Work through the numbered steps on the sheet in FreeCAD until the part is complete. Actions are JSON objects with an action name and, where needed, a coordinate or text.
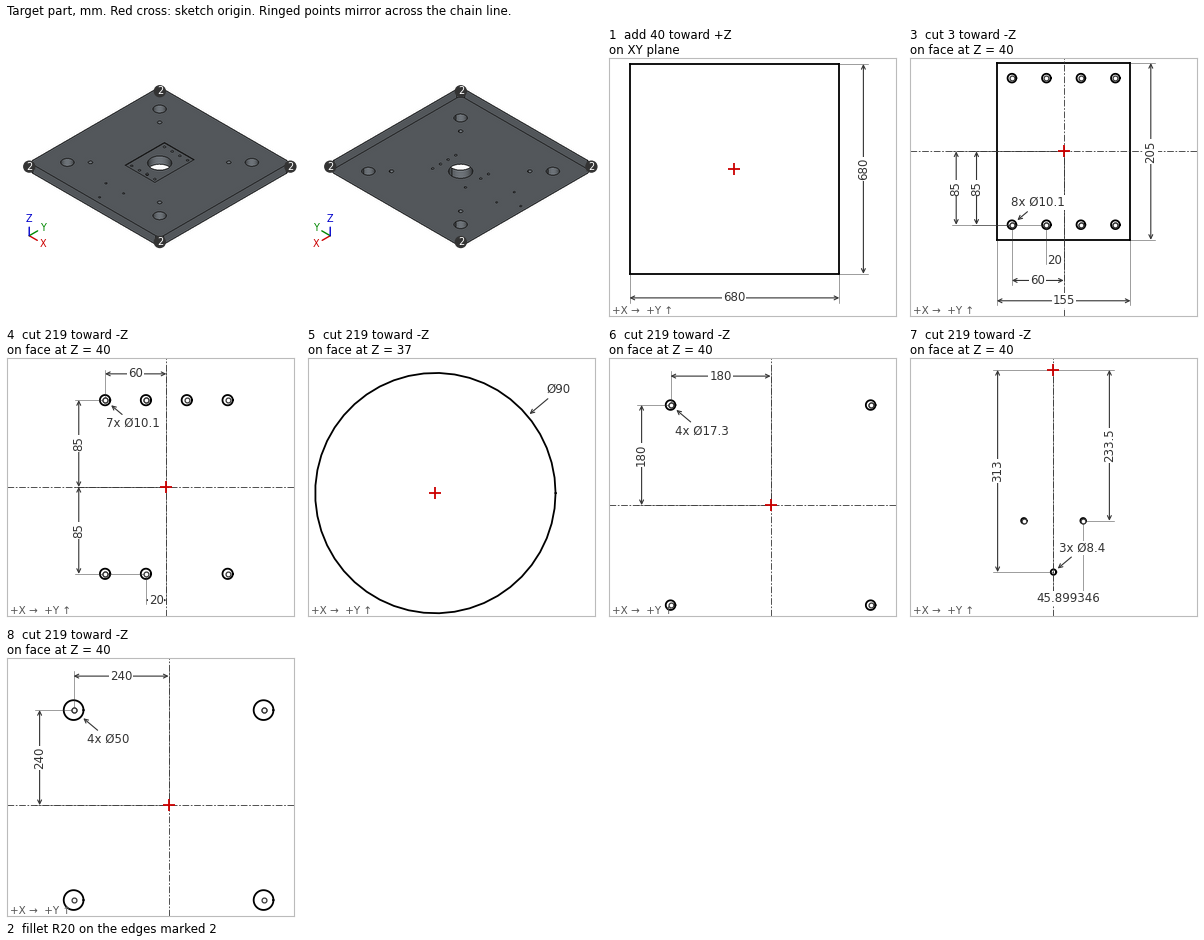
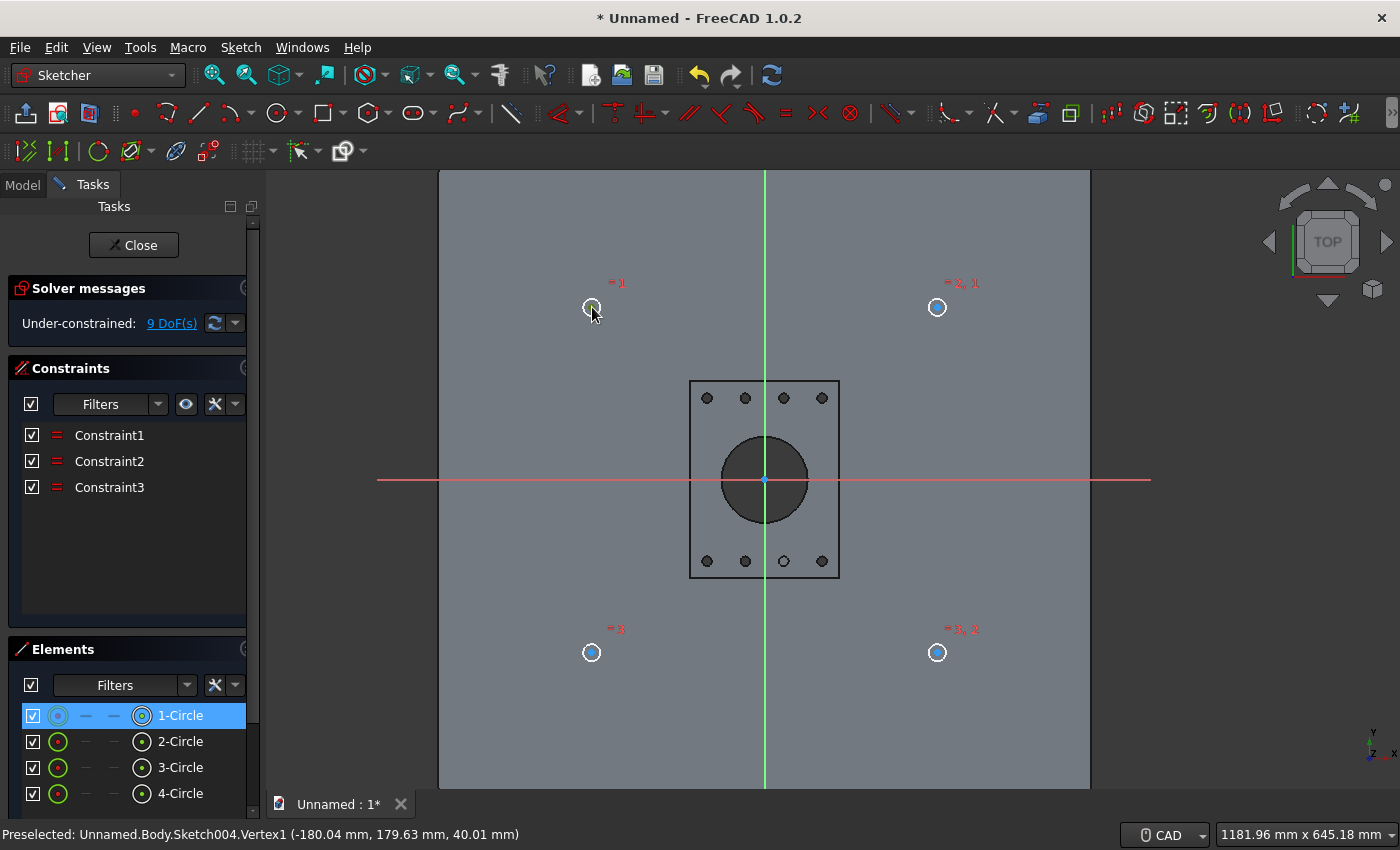
{"action": "left_click", "coordinate": [937, 307]}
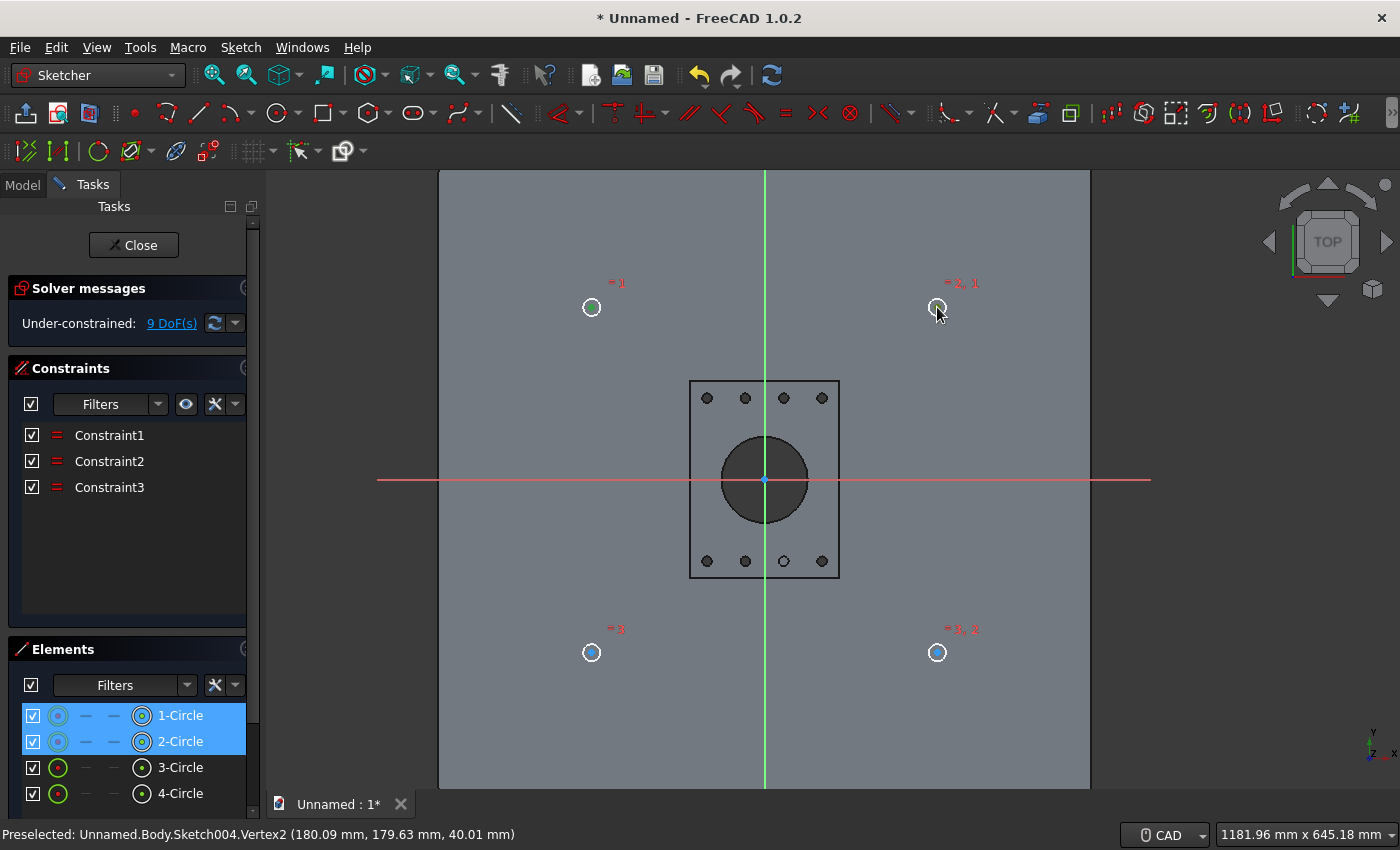
{"action": "left_click", "coordinate": [765, 721]}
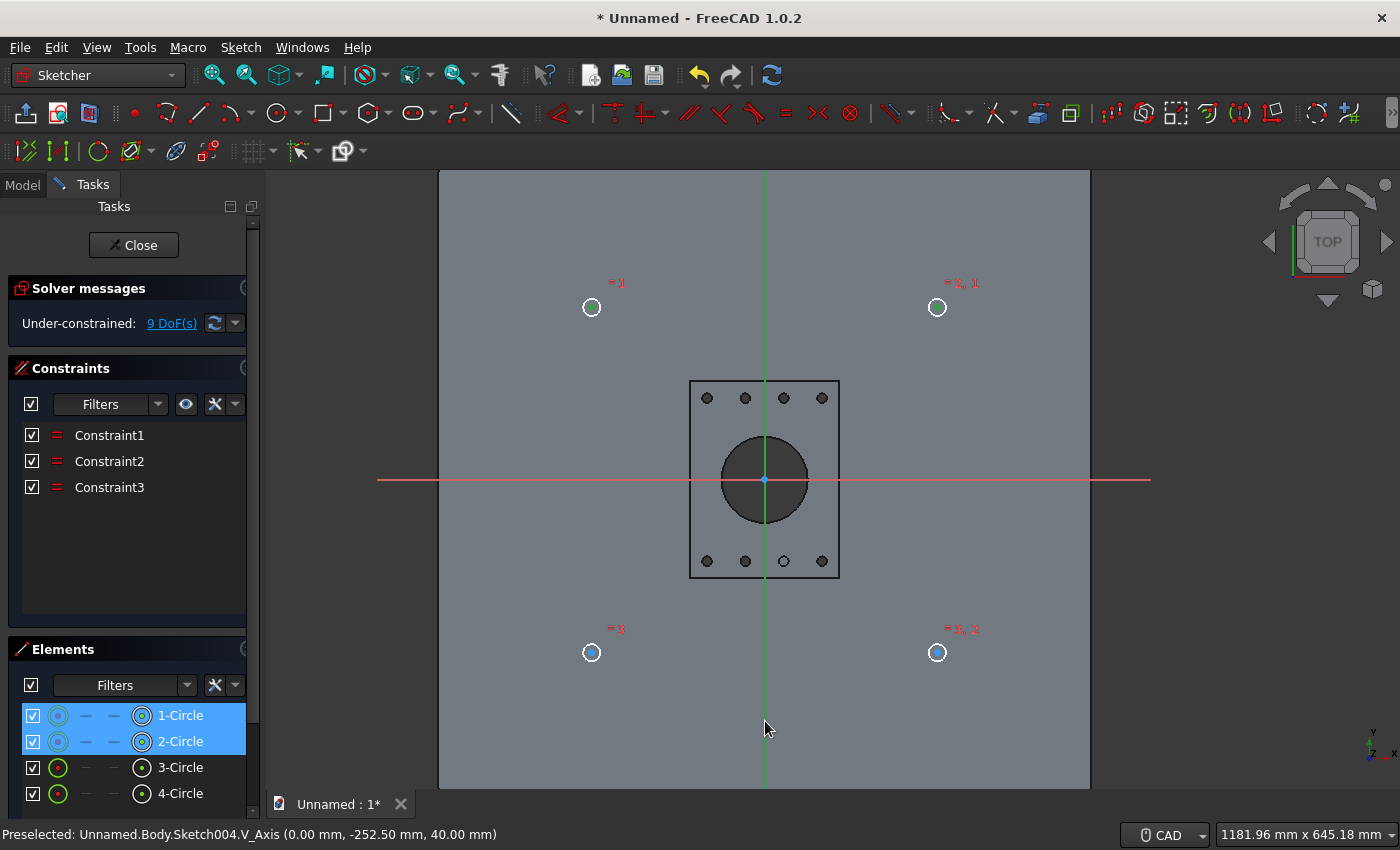
{"action": "left_click", "coordinate": [818, 114]}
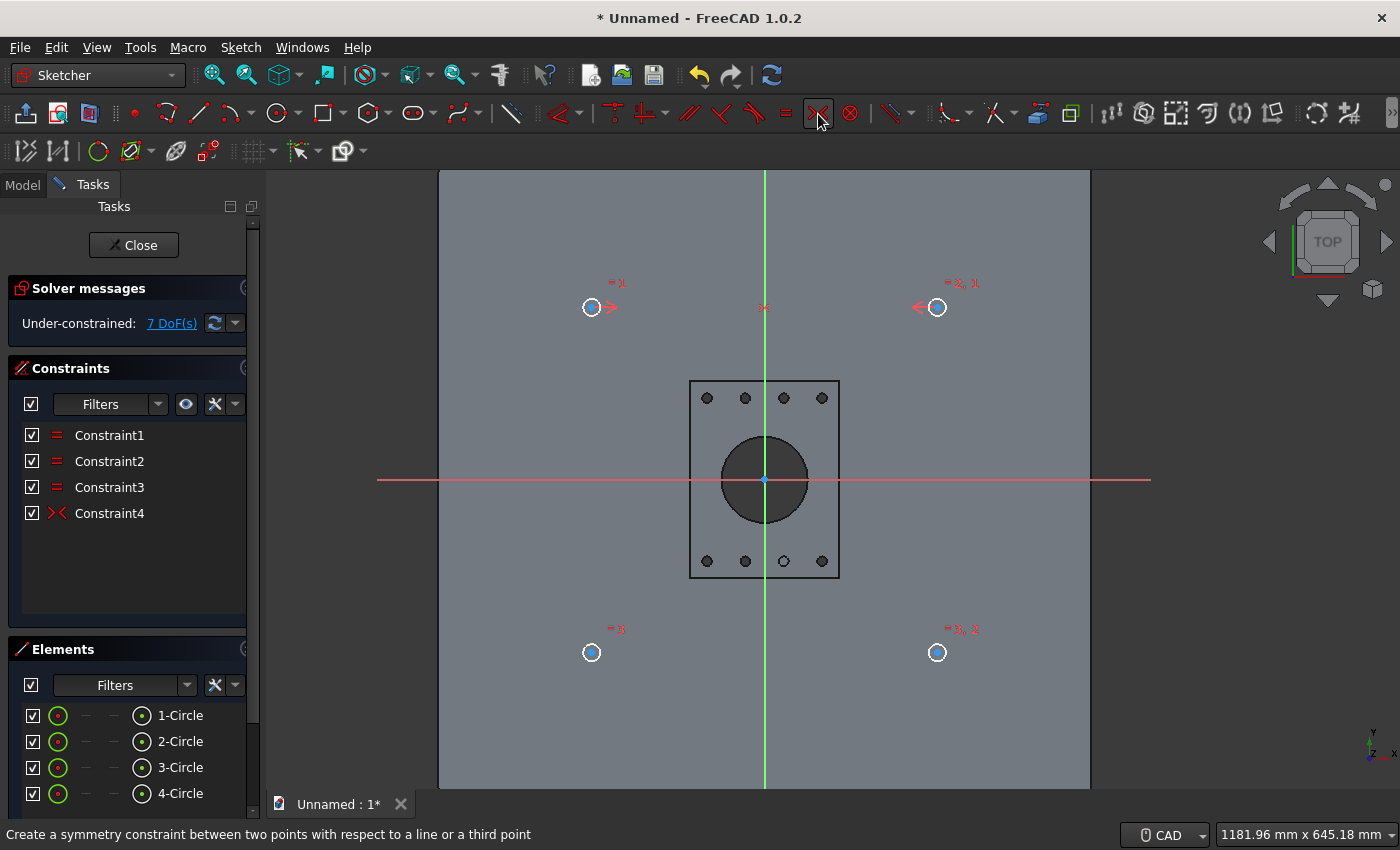
{"action": "left_click", "coordinate": [937, 307]}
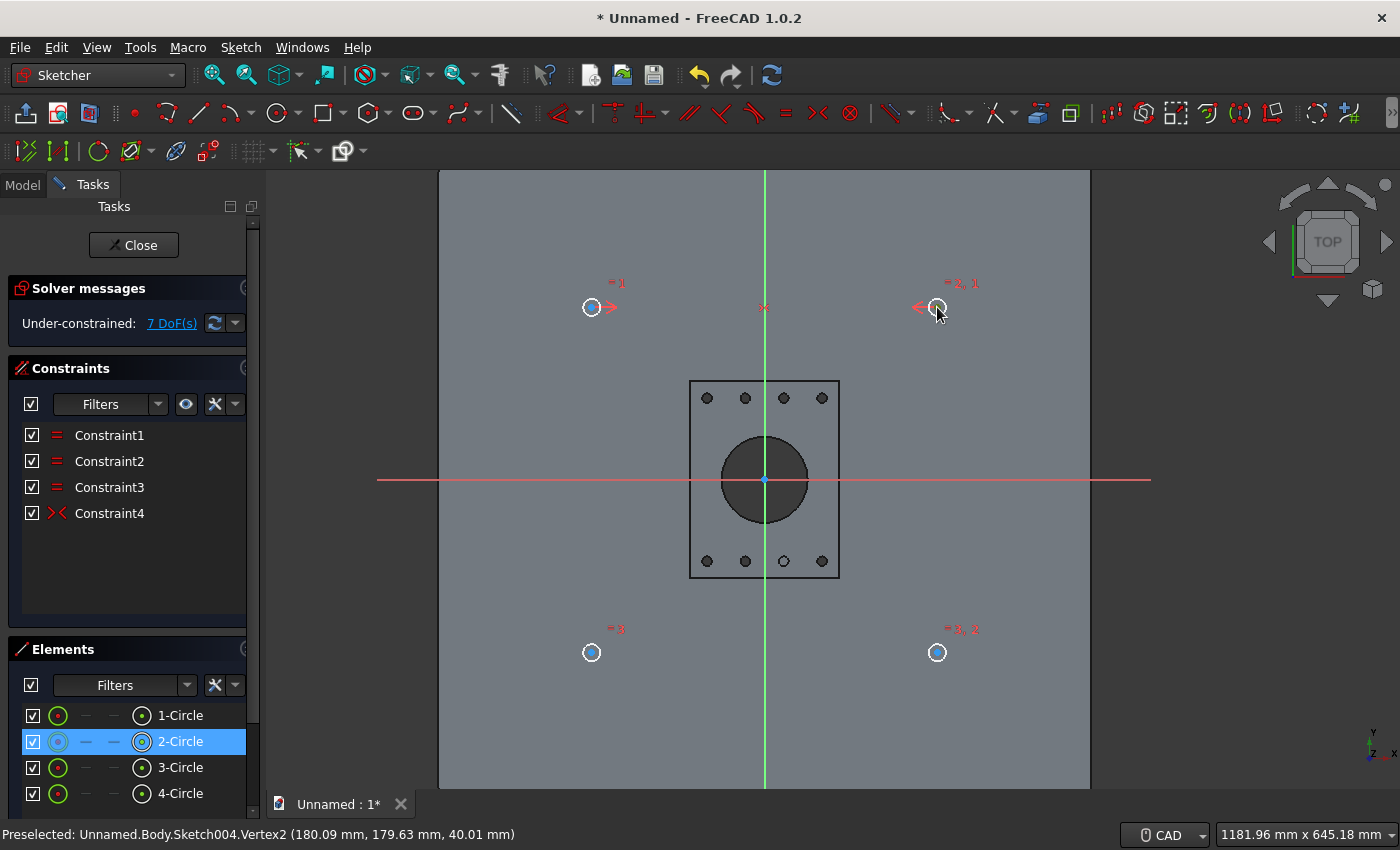
{"action": "left_click", "coordinate": [937, 653]}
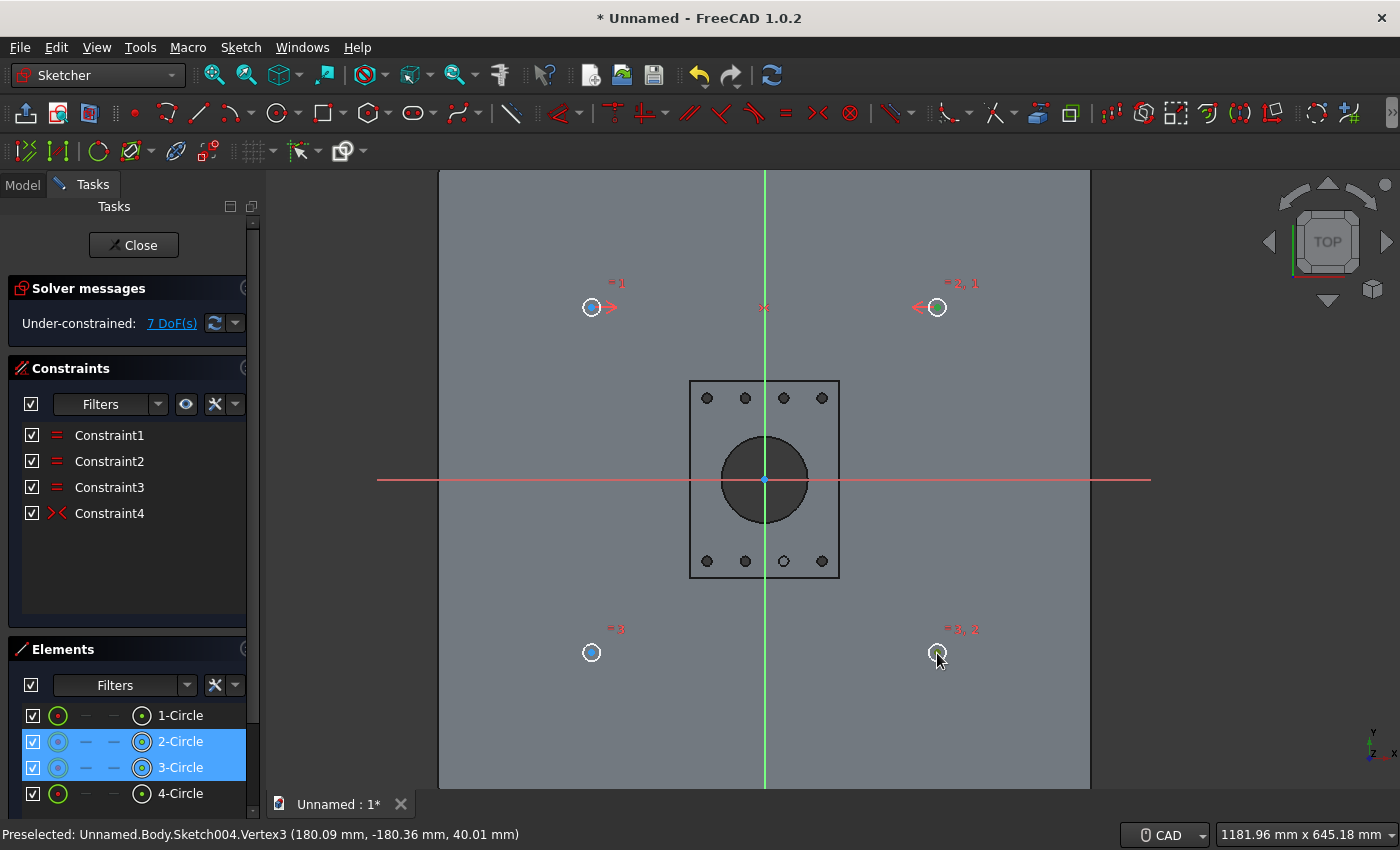
{"action": "left_click", "coordinate": [428, 480]}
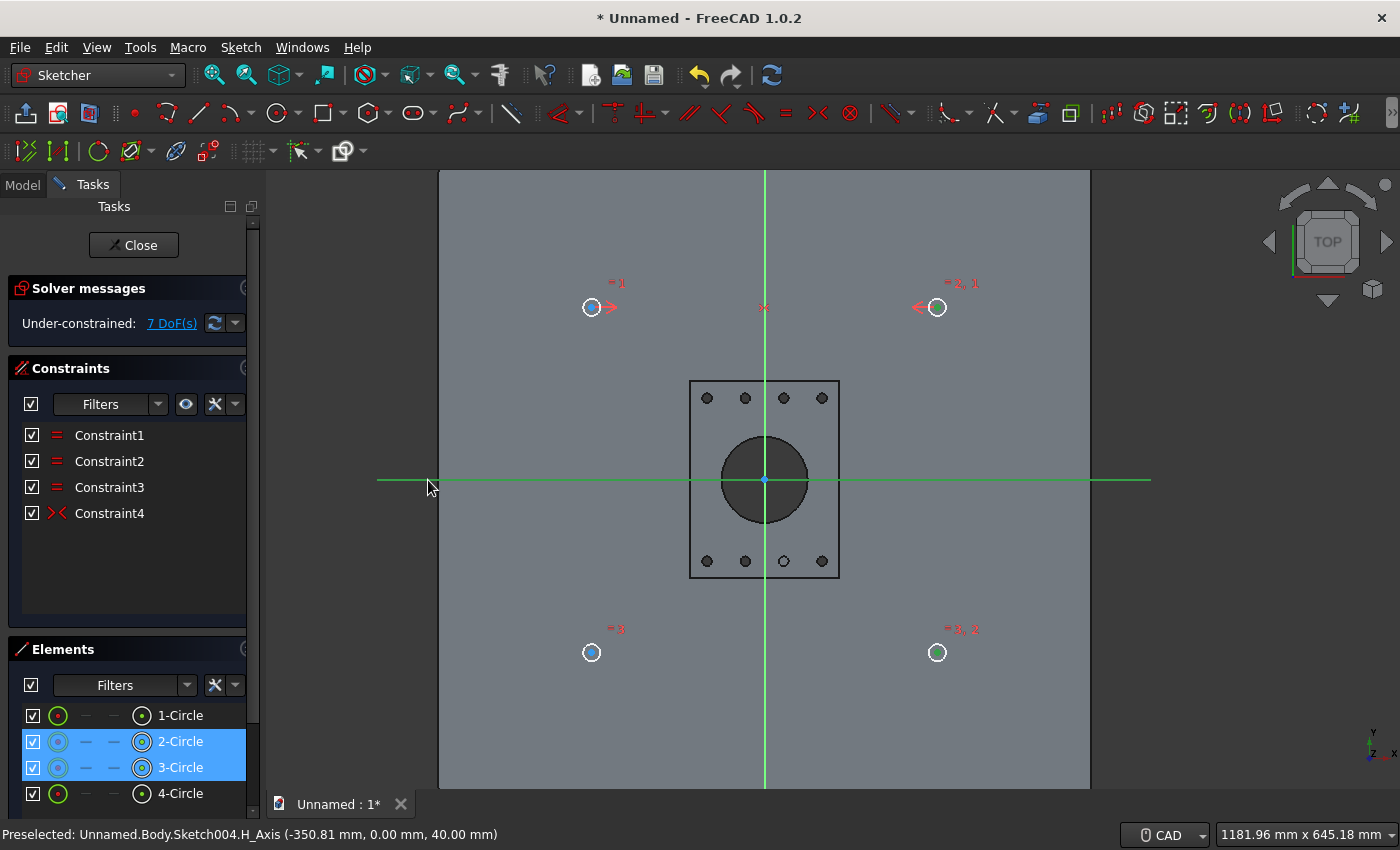
{"action": "left_click", "coordinate": [818, 114]}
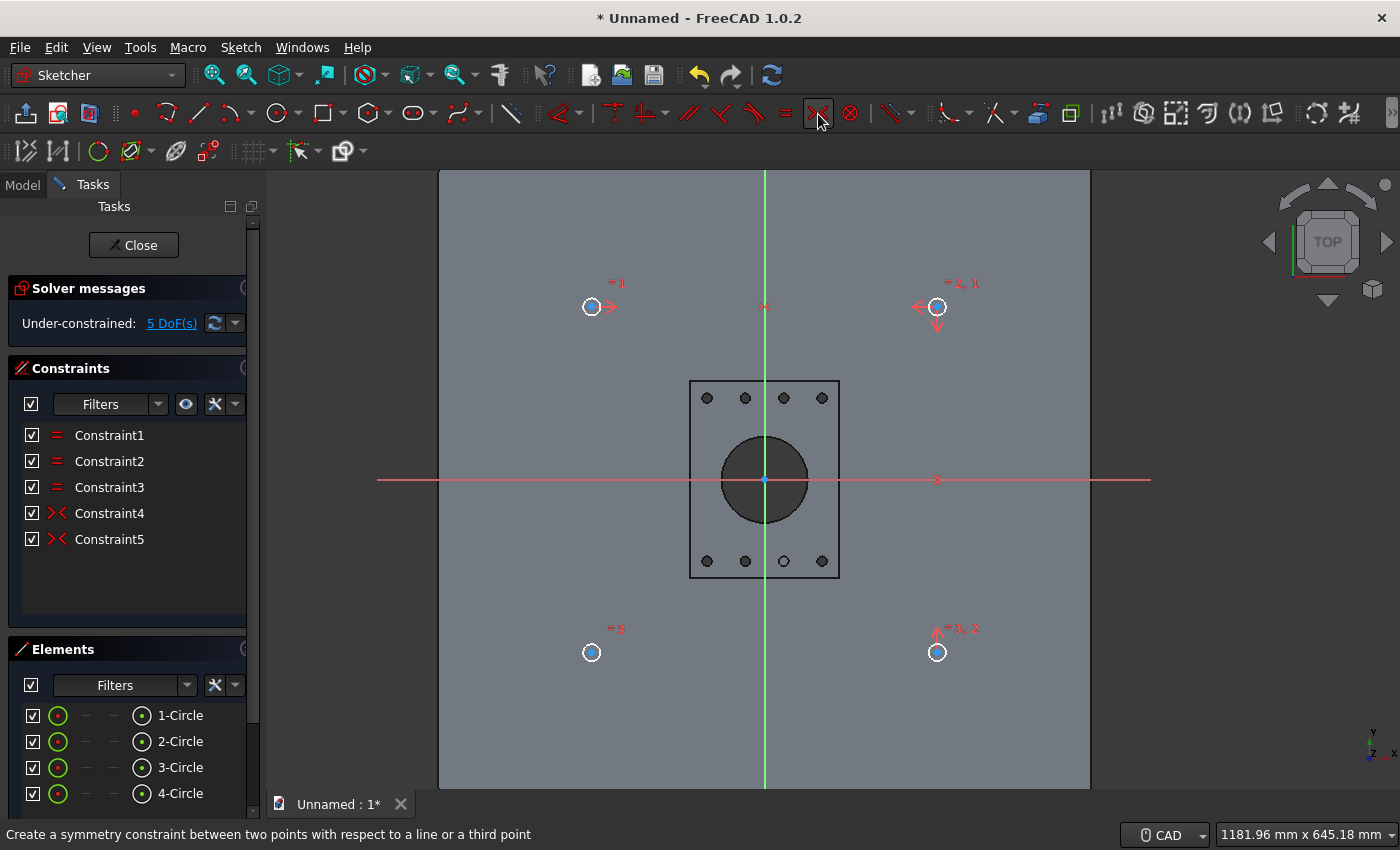
{"action": "left_click", "coordinate": [592, 307]}